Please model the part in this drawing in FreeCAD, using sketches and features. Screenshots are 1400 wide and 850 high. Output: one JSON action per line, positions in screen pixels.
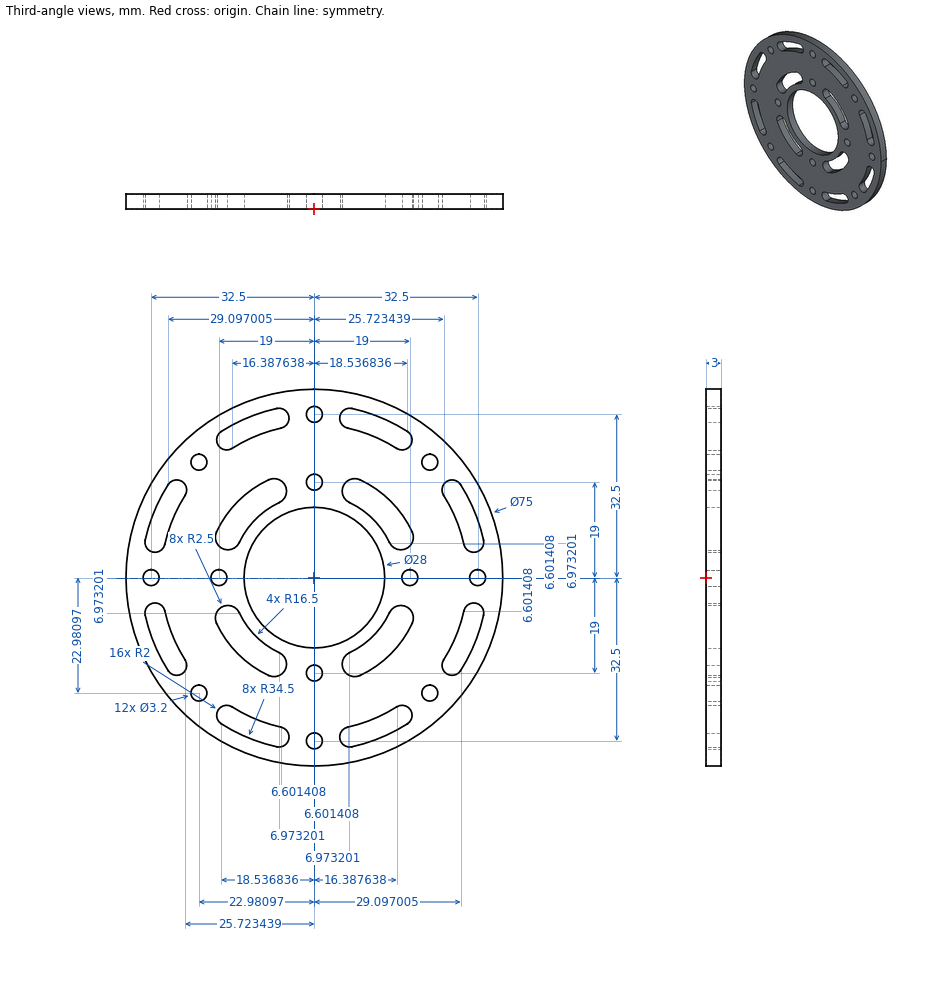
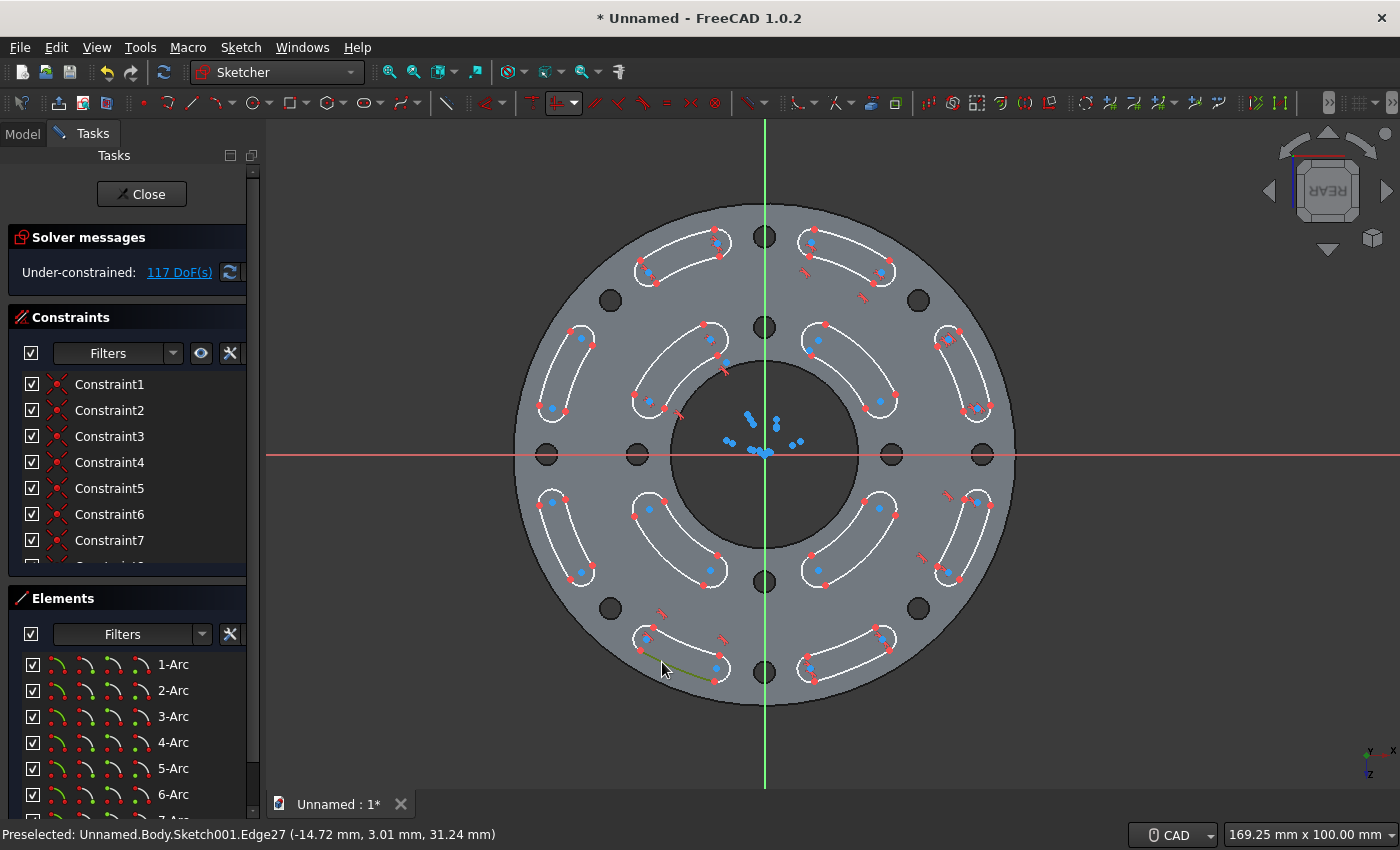
{"action": "left_click", "coordinate": [726, 678]}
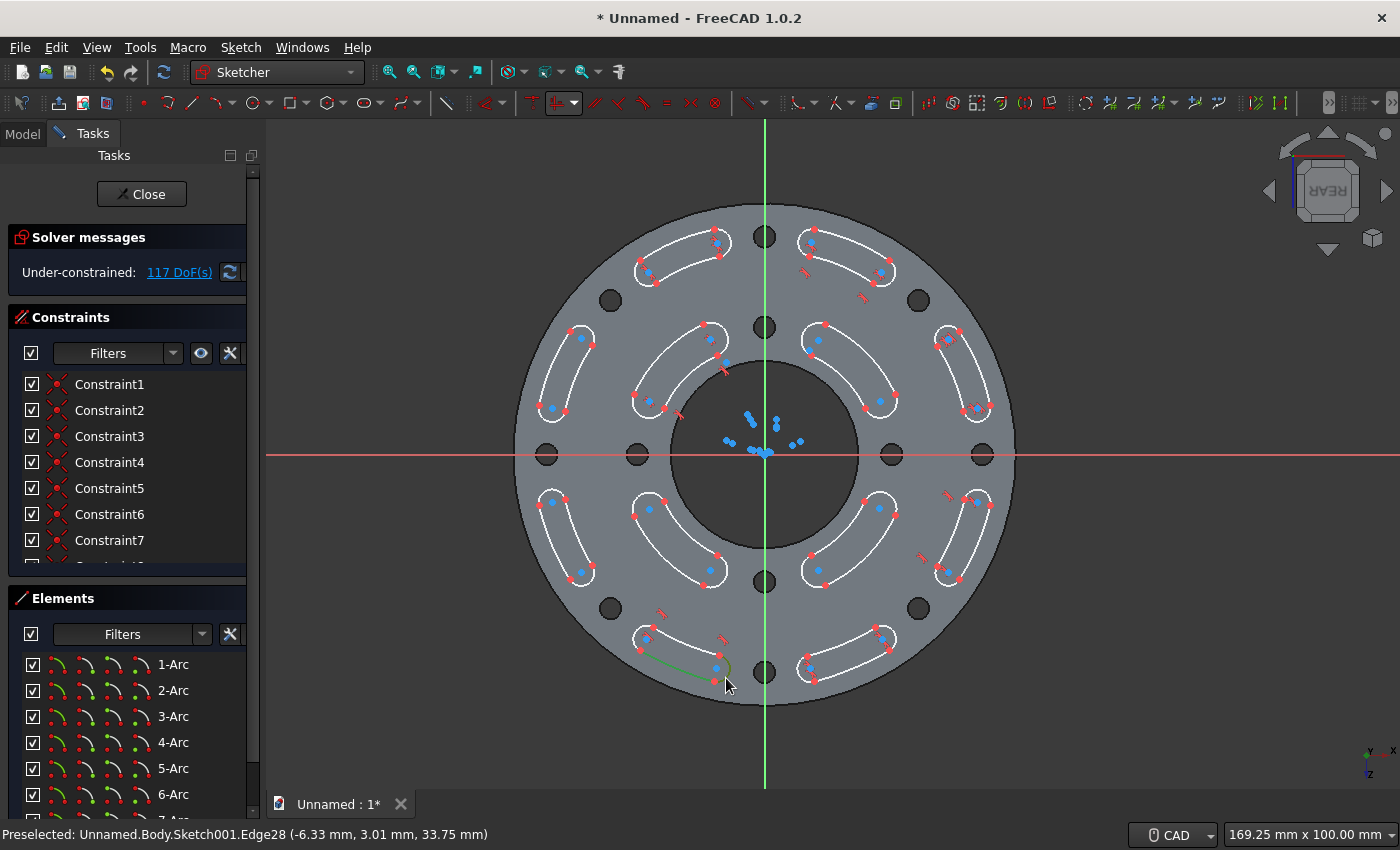
{"action": "left_click", "coordinate": [644, 104]}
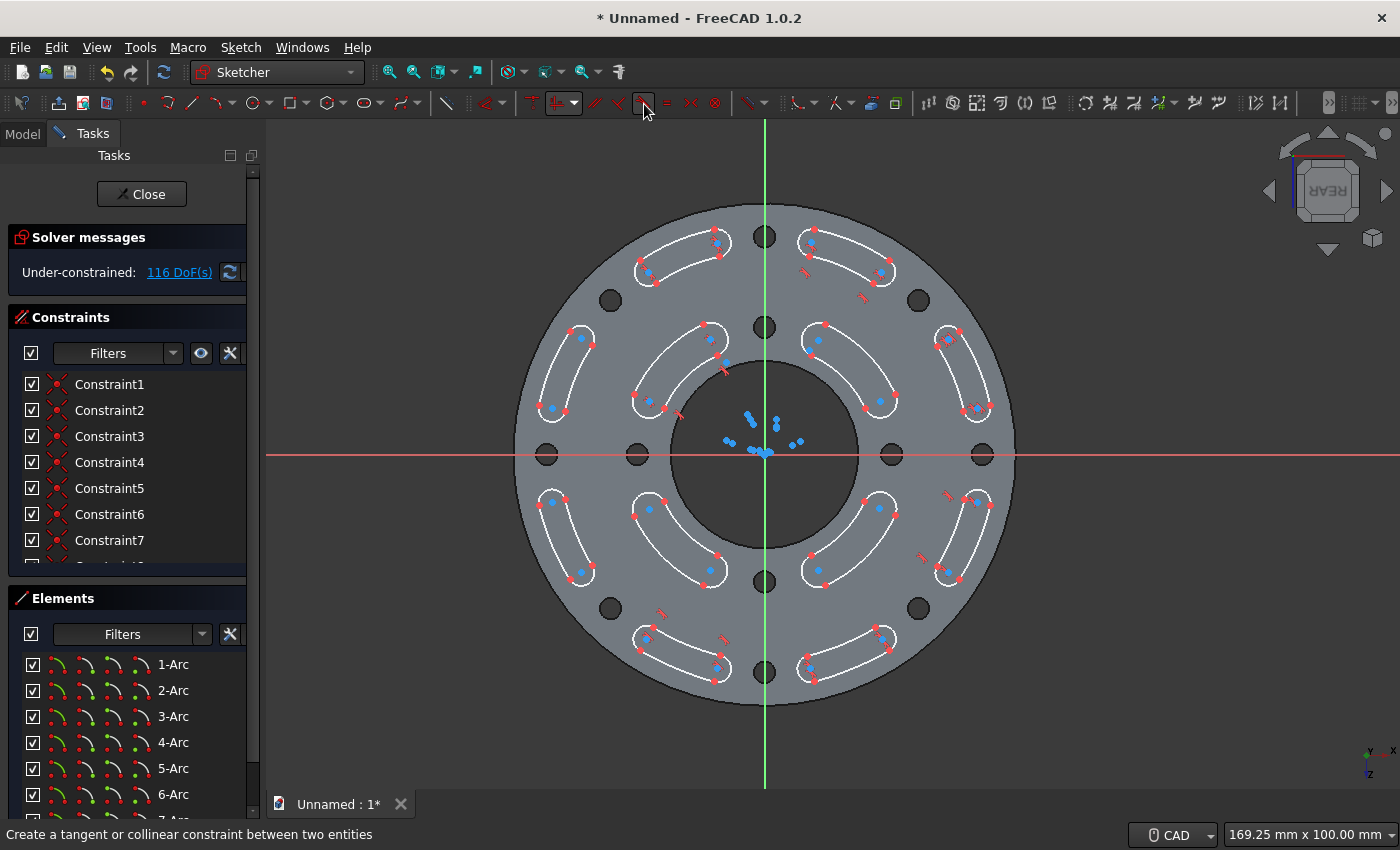
{"action": "left_click", "coordinate": [557, 491]}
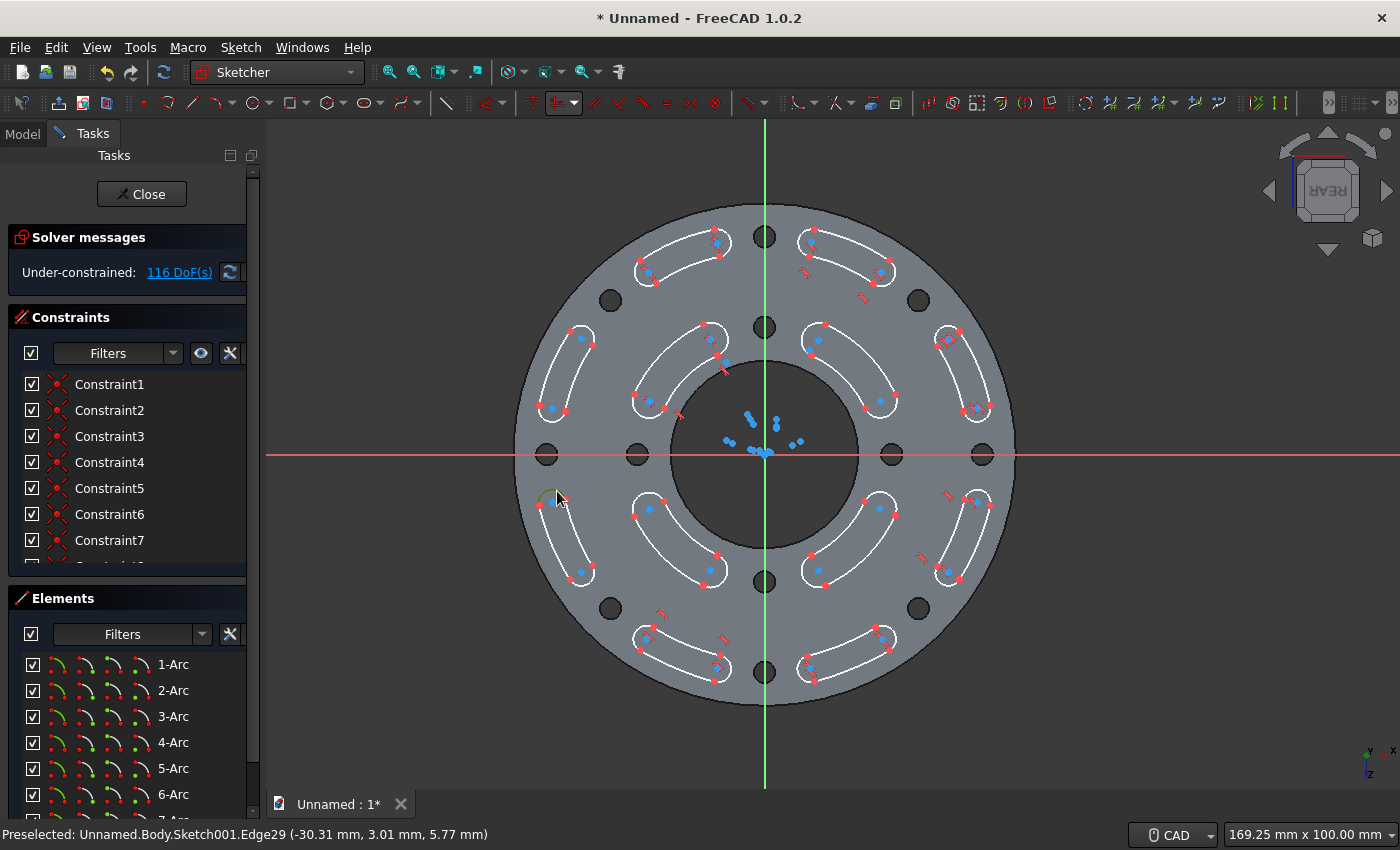
{"action": "left_click", "coordinate": [546, 529]}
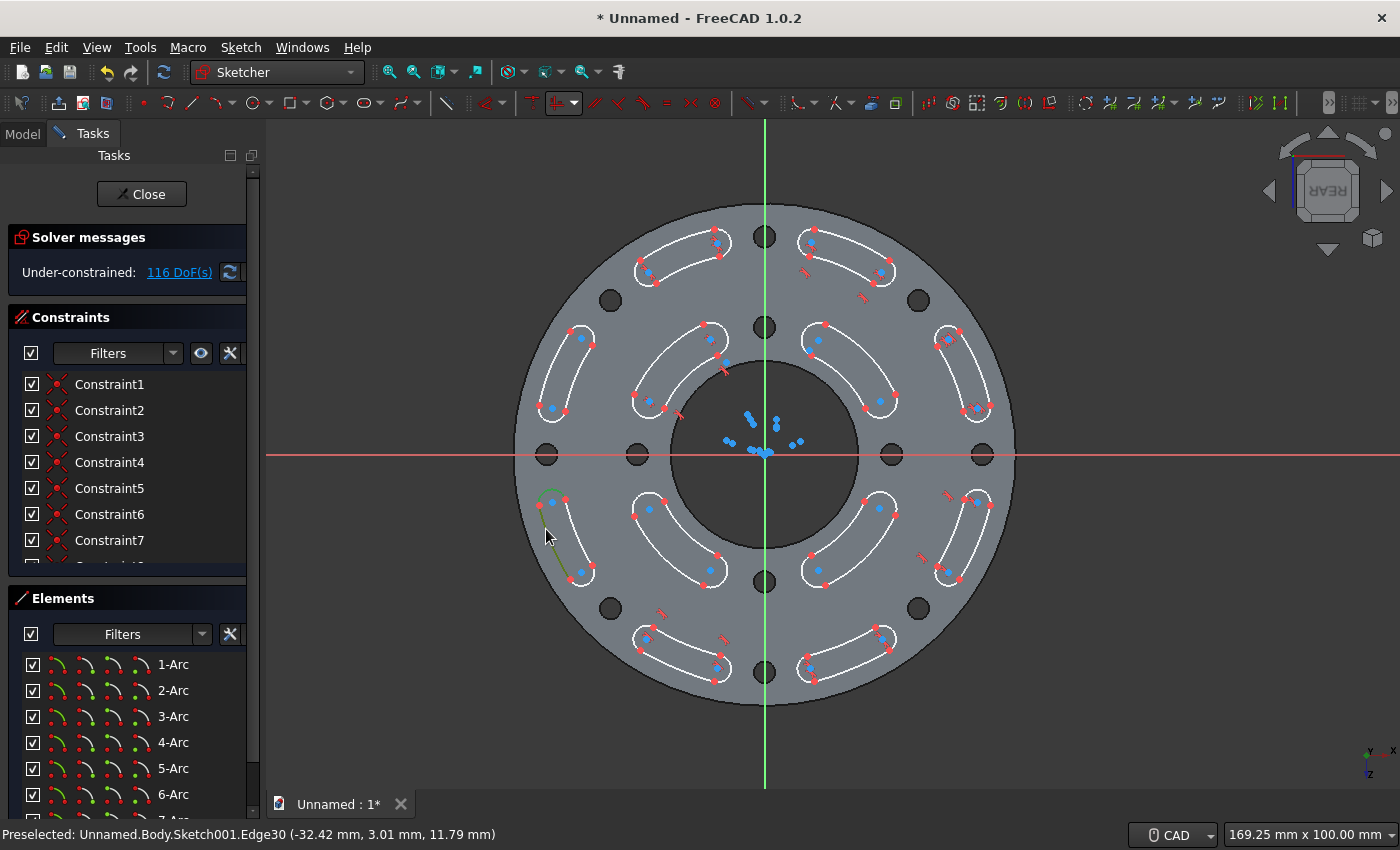
{"action": "left_click", "coordinate": [644, 104]}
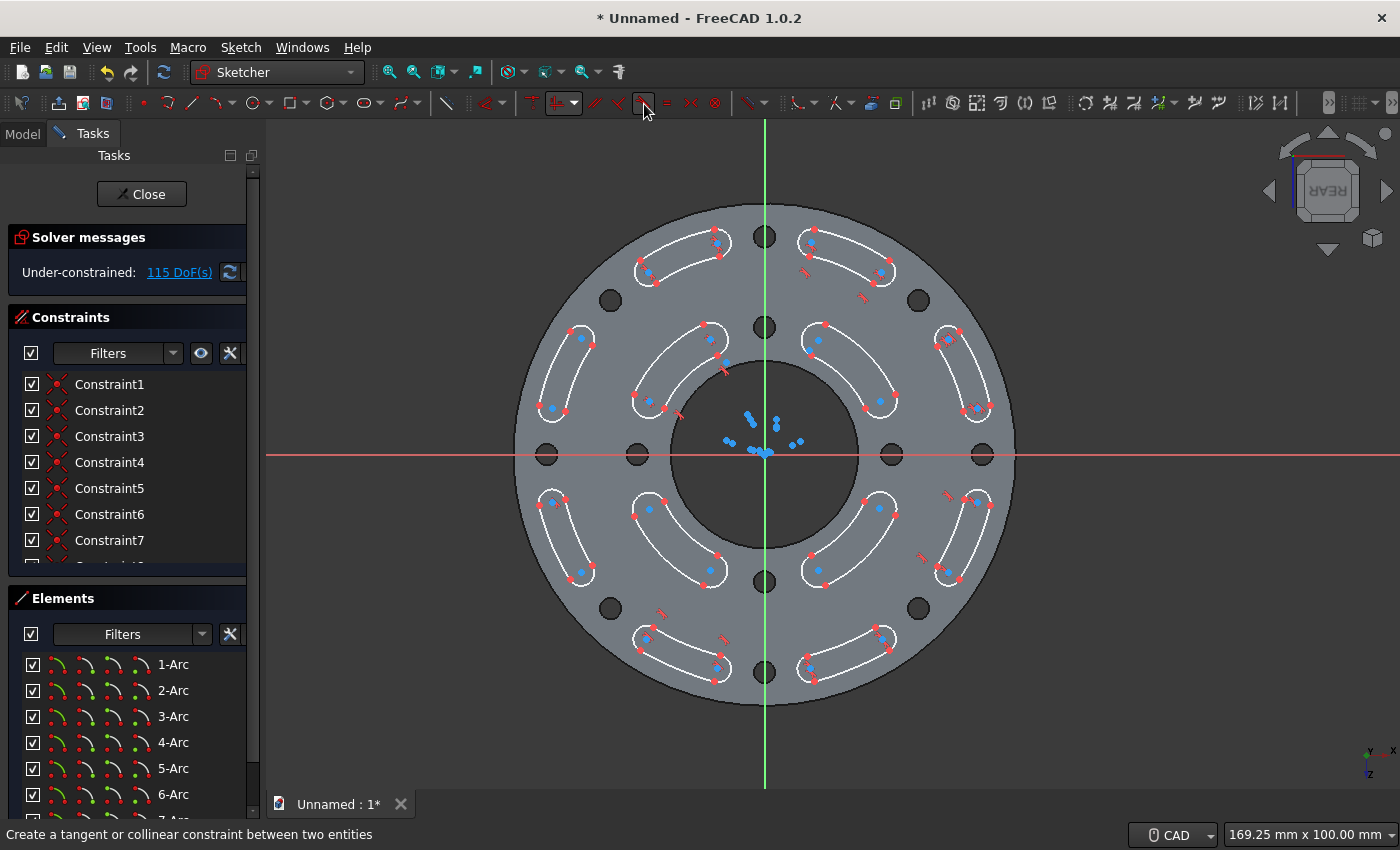
{"action": "left_click", "coordinate": [557, 491]}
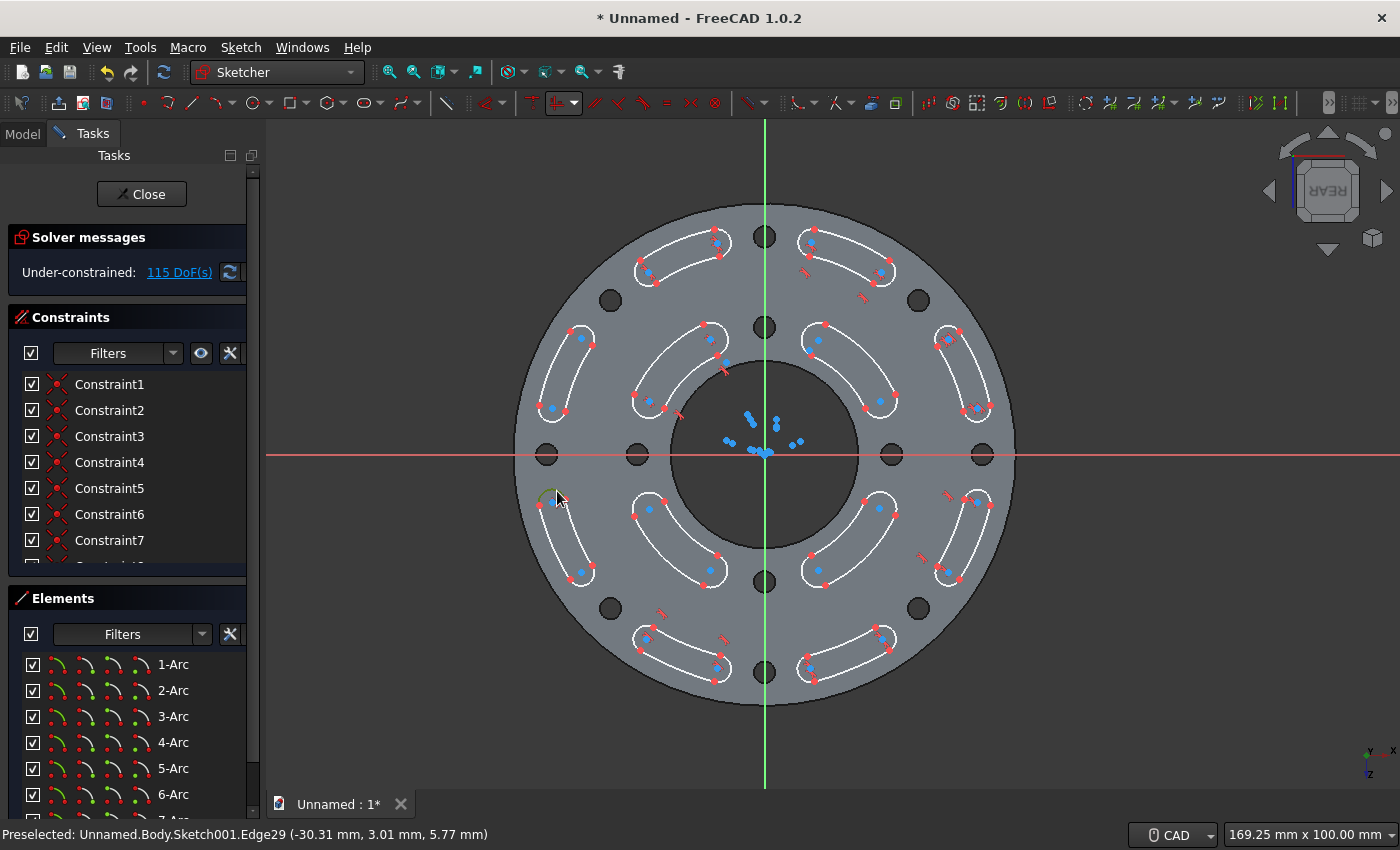
{"action": "left_click", "coordinate": [571, 520]}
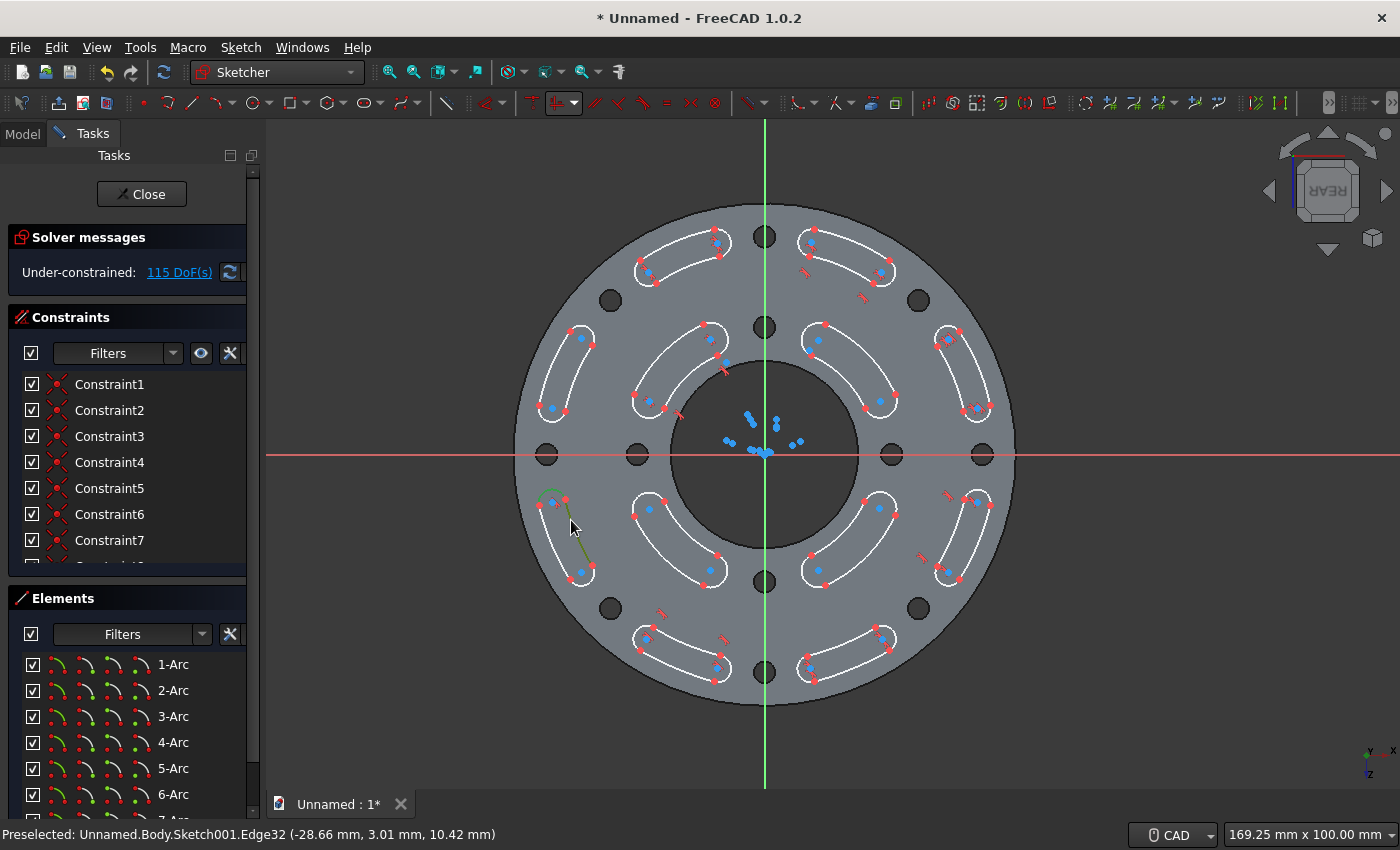
{"action": "left_click", "coordinate": [644, 104]}